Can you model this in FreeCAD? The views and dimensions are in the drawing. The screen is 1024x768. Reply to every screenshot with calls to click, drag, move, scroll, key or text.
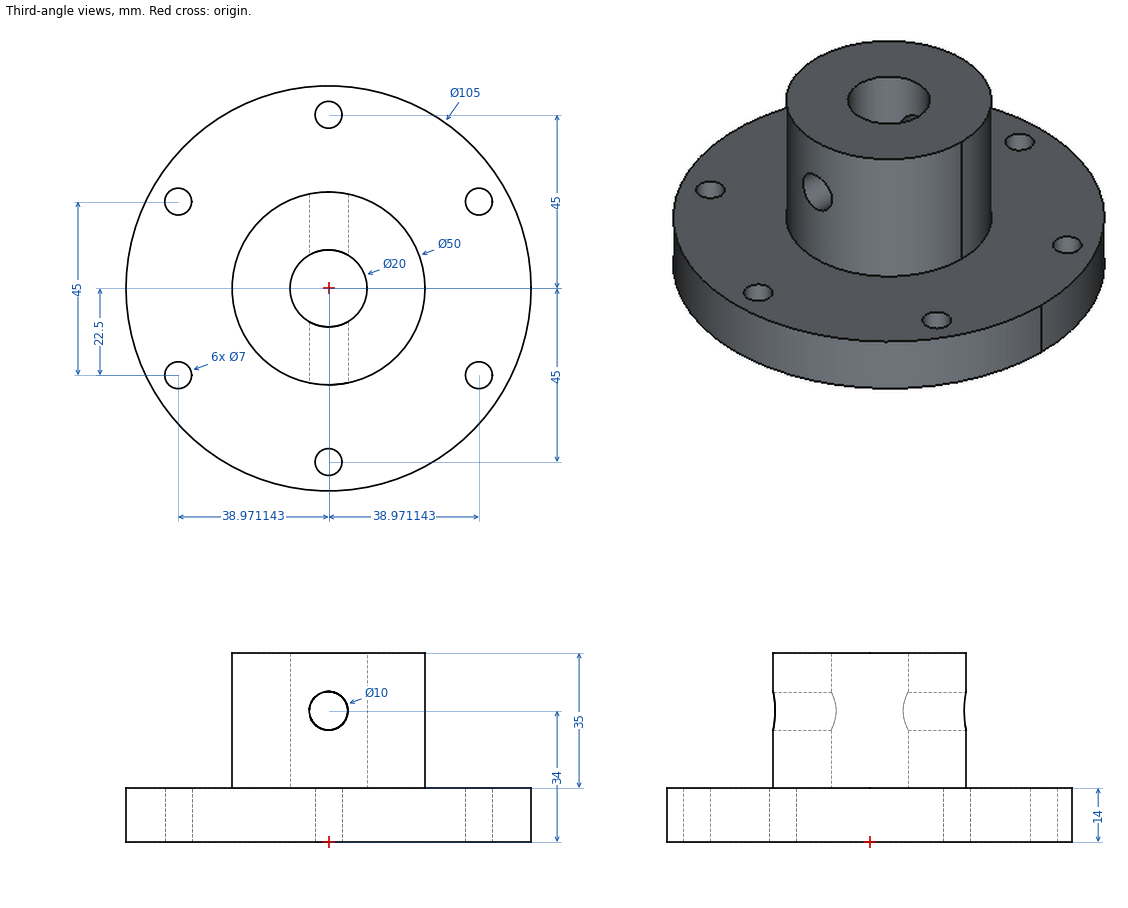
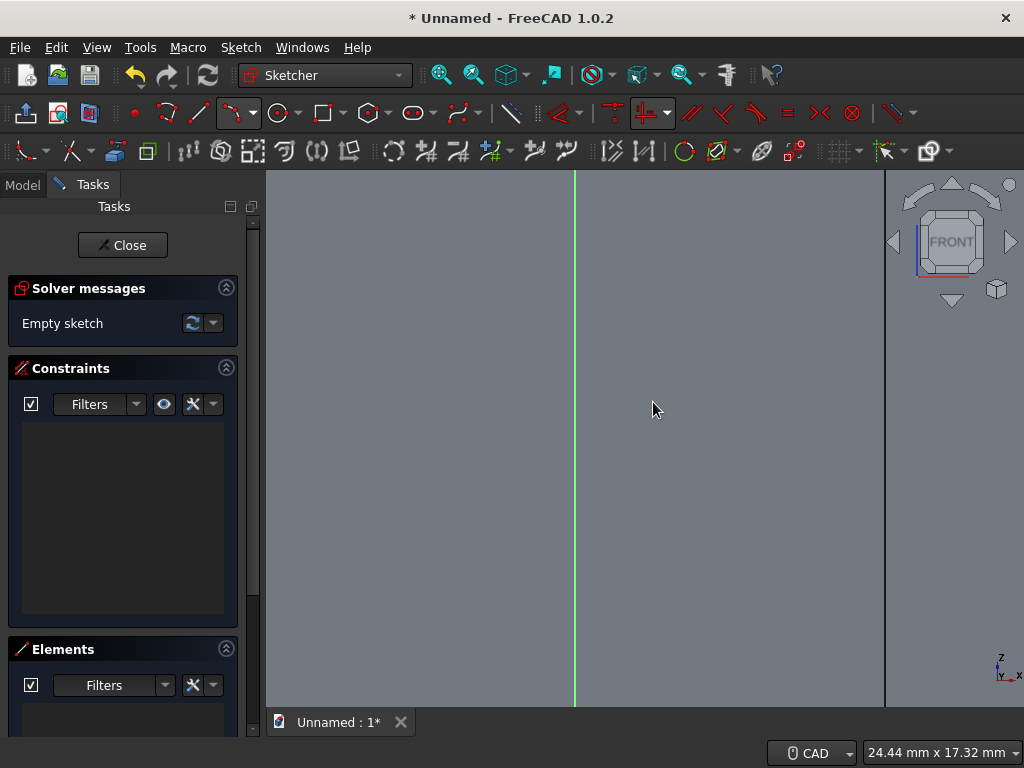
key(g)
key(c)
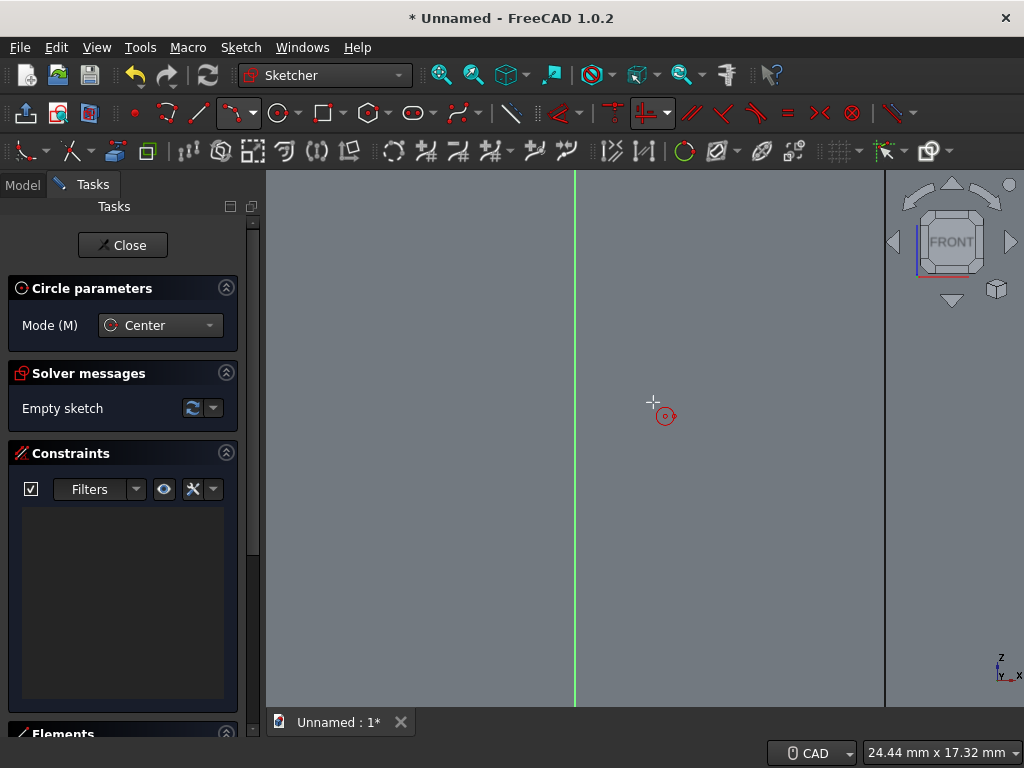
click(575, 433)
move(685, 324)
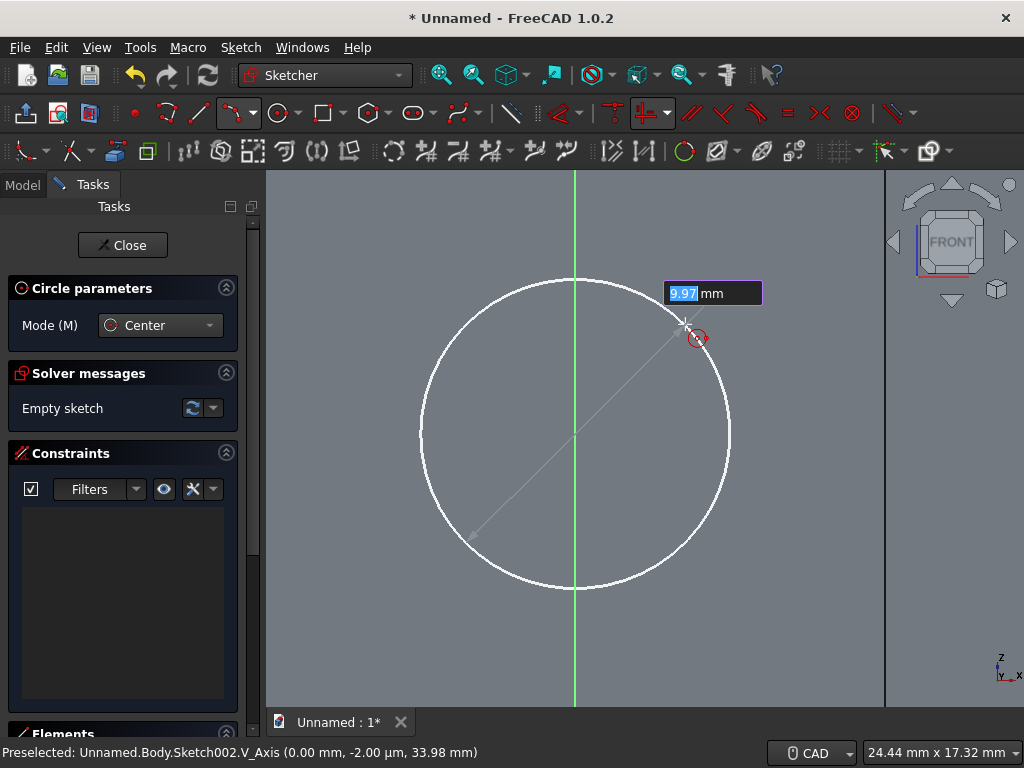
text(10)
key(Return)
key(Escape)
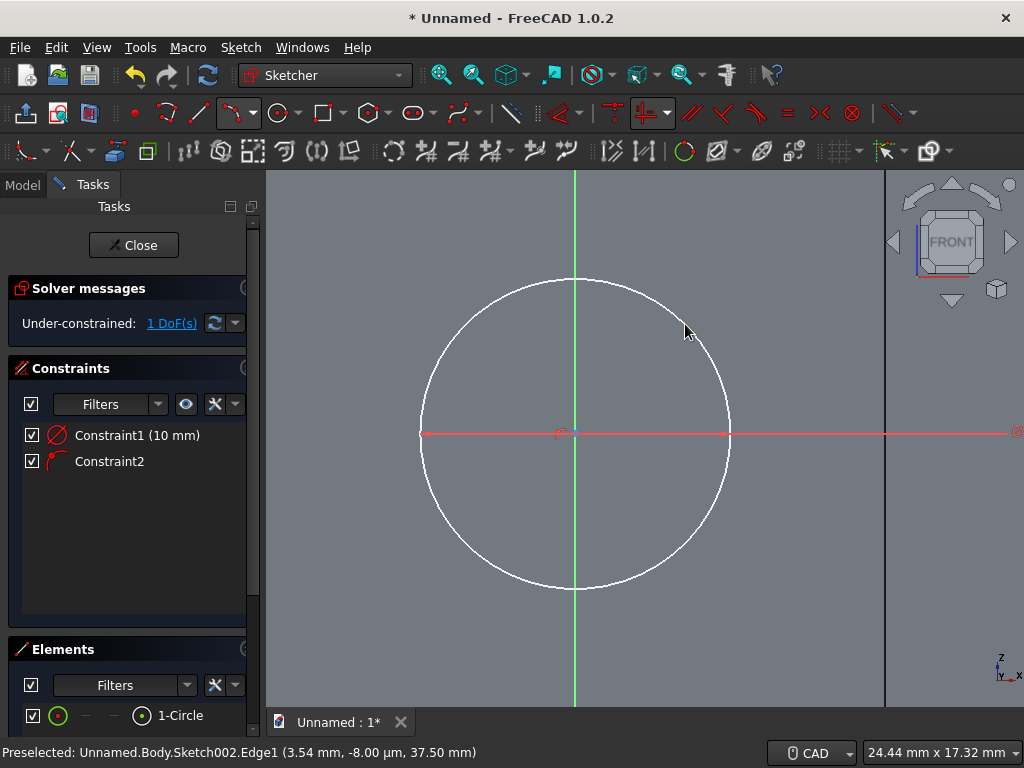
key(d)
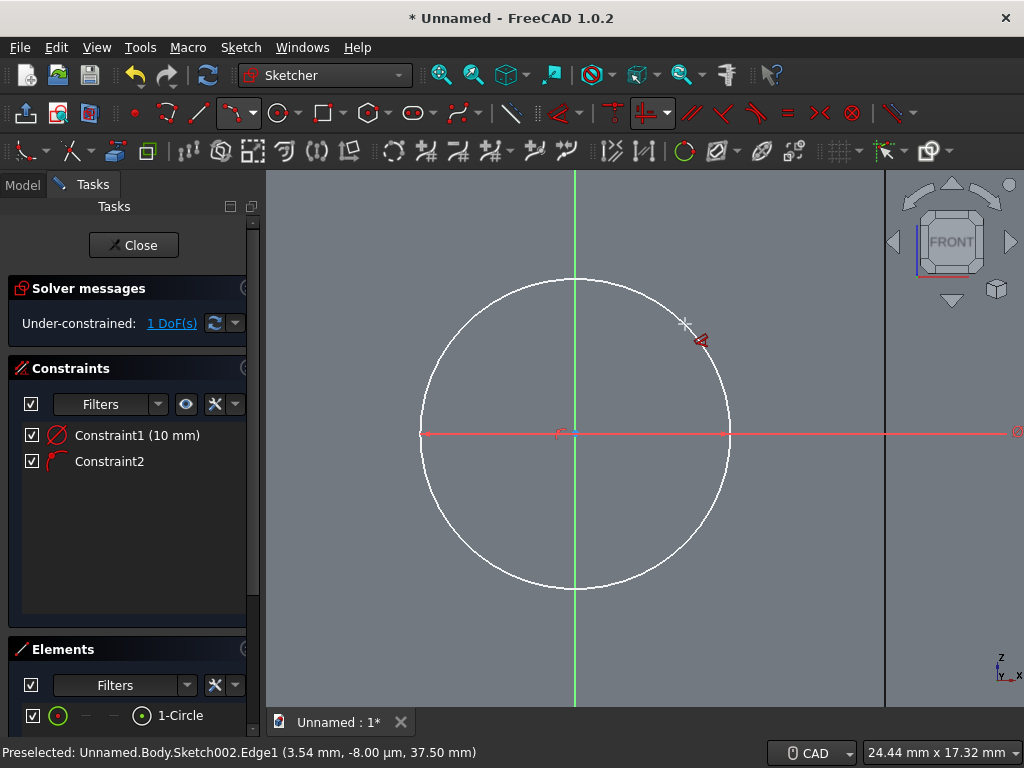
click(575, 434)
click(609, 556)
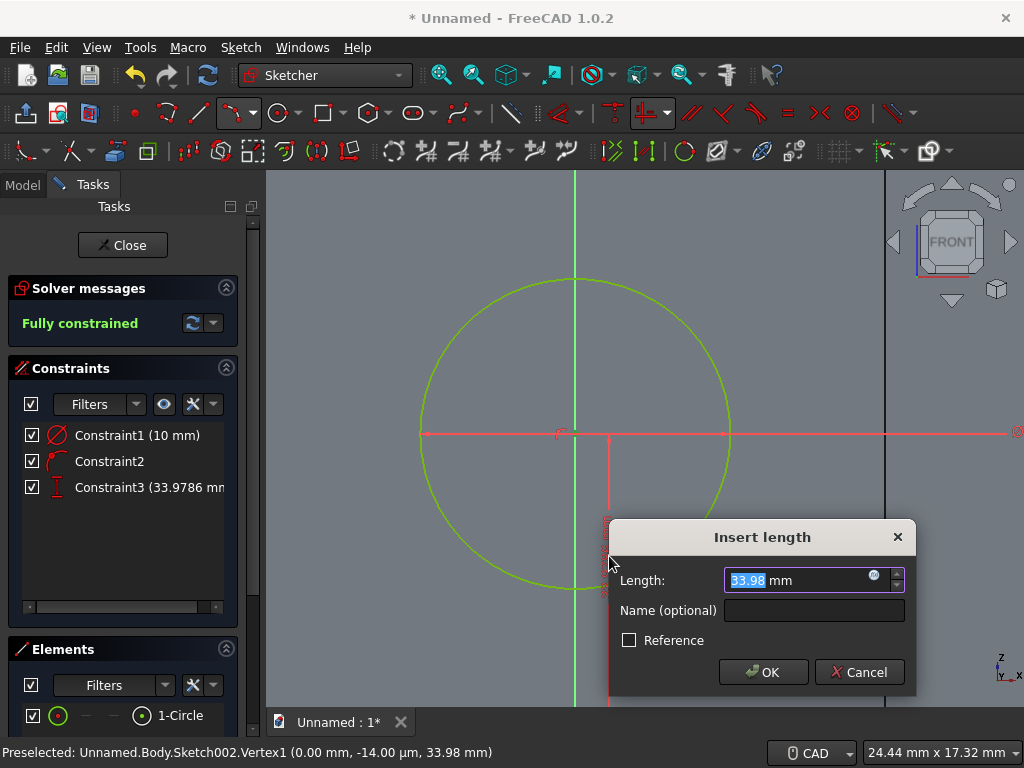
text(34)
key(Return)
key(Escape)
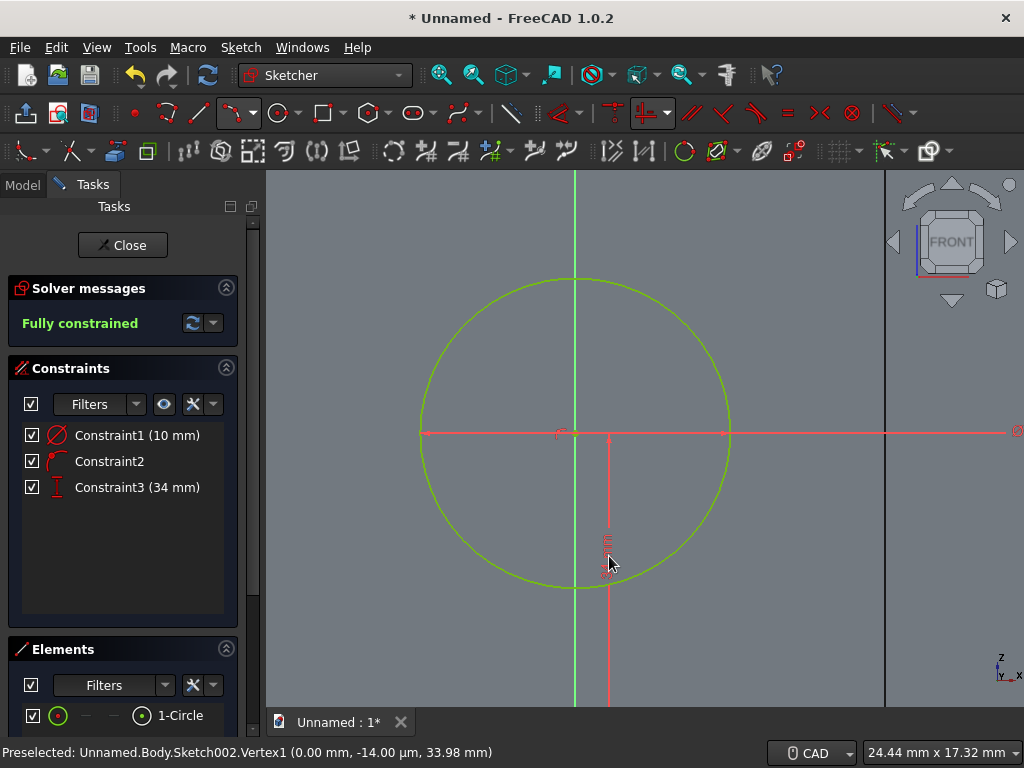
click(123, 245)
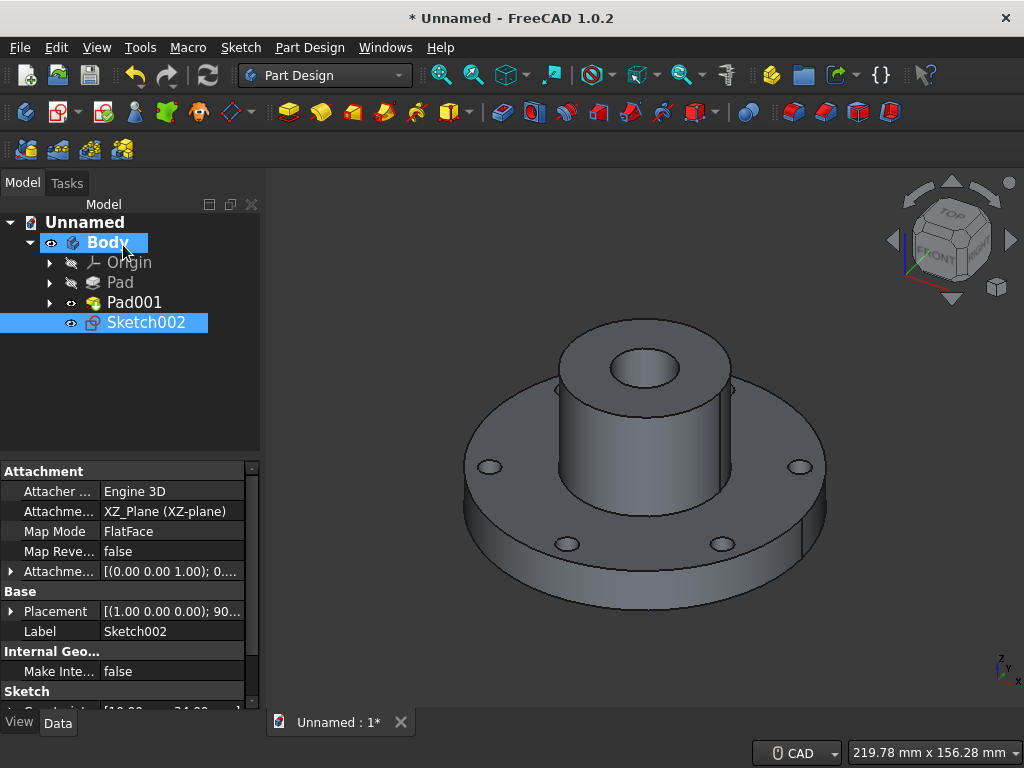
click(504, 112)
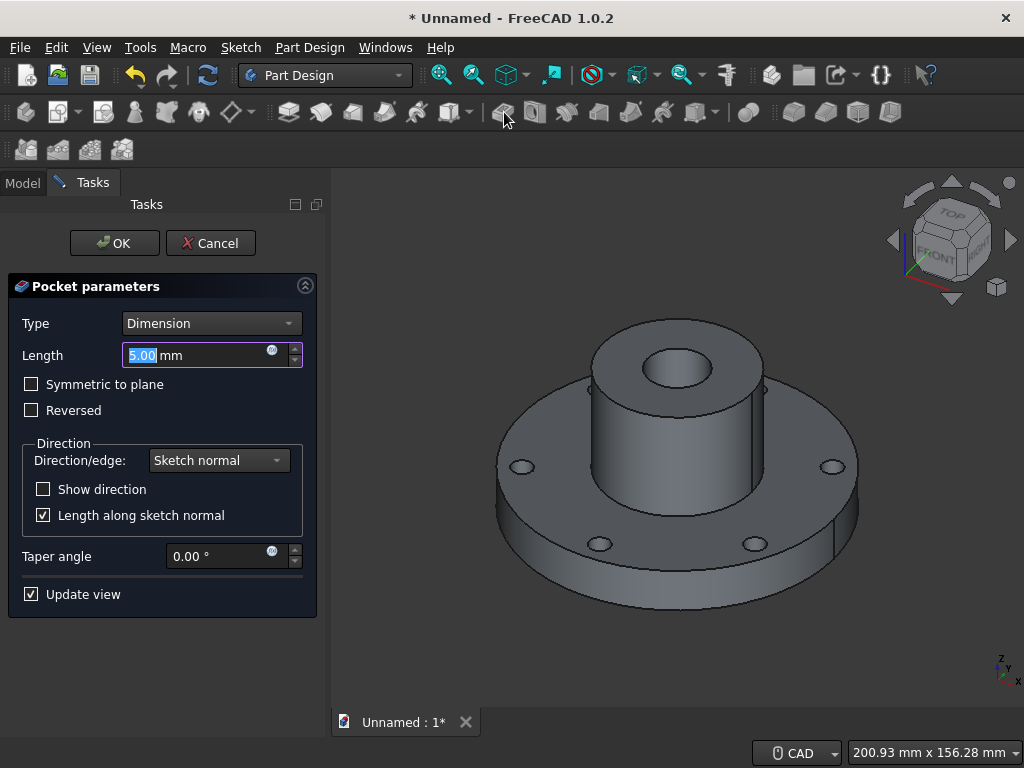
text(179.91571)
key(Tab)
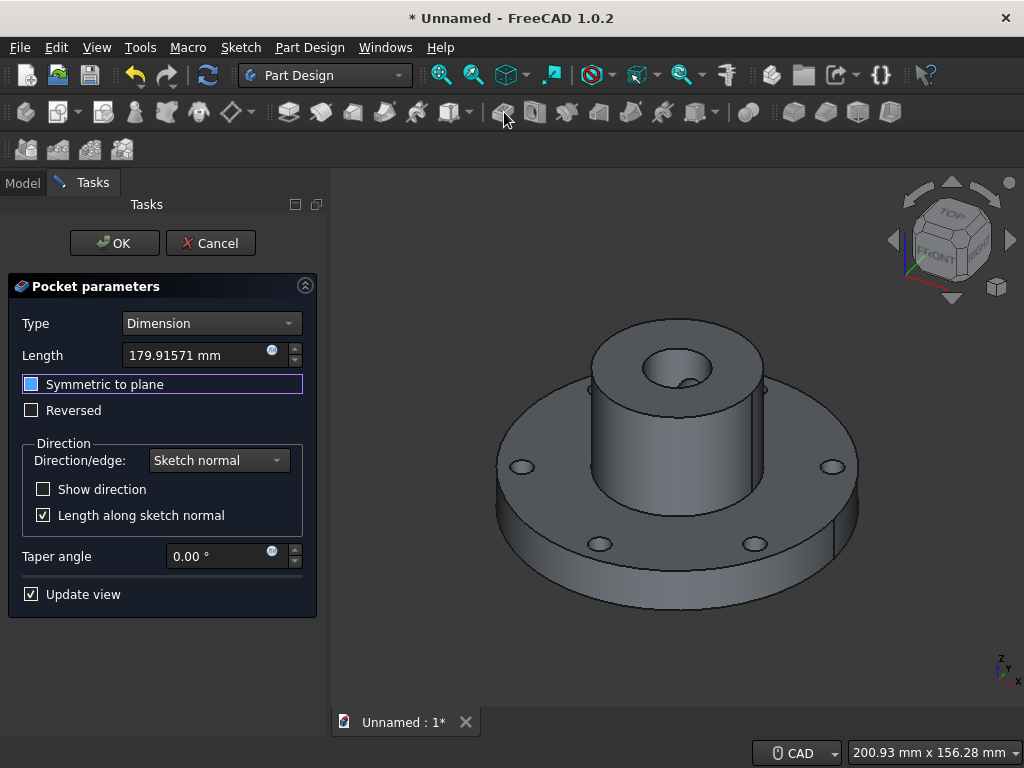
click(30, 384)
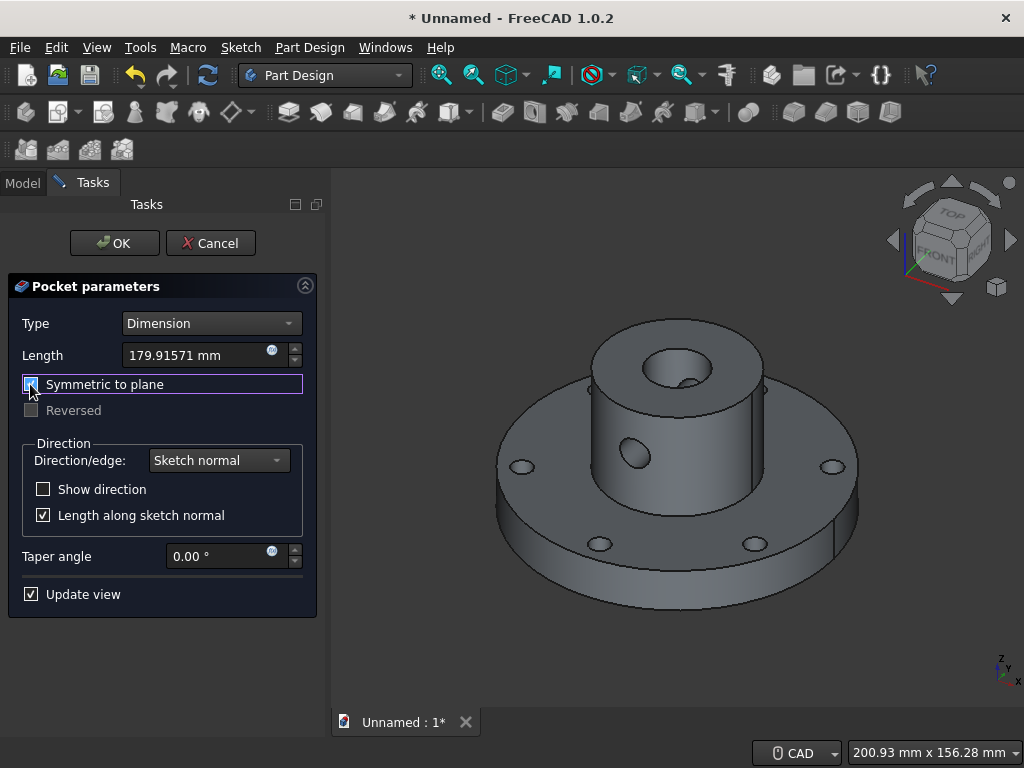
click(115, 243)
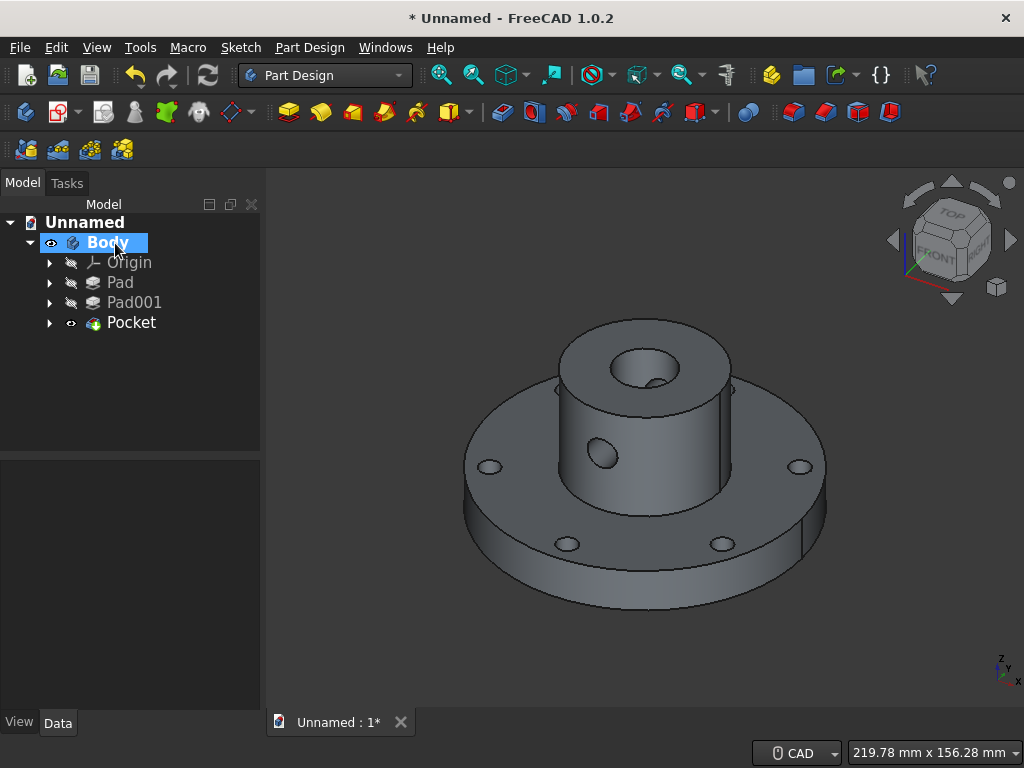
key(0)